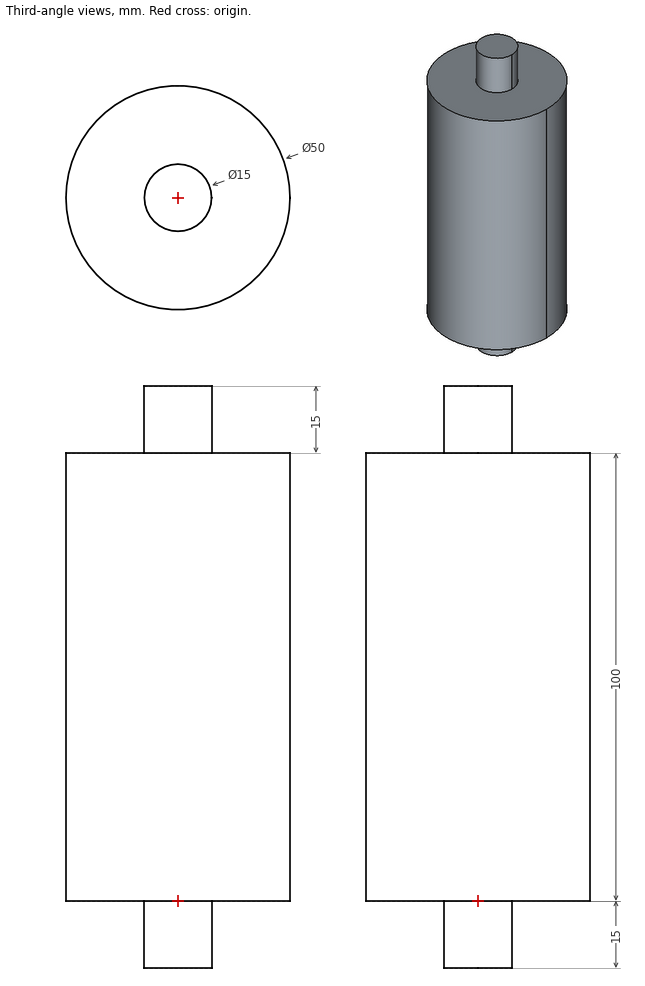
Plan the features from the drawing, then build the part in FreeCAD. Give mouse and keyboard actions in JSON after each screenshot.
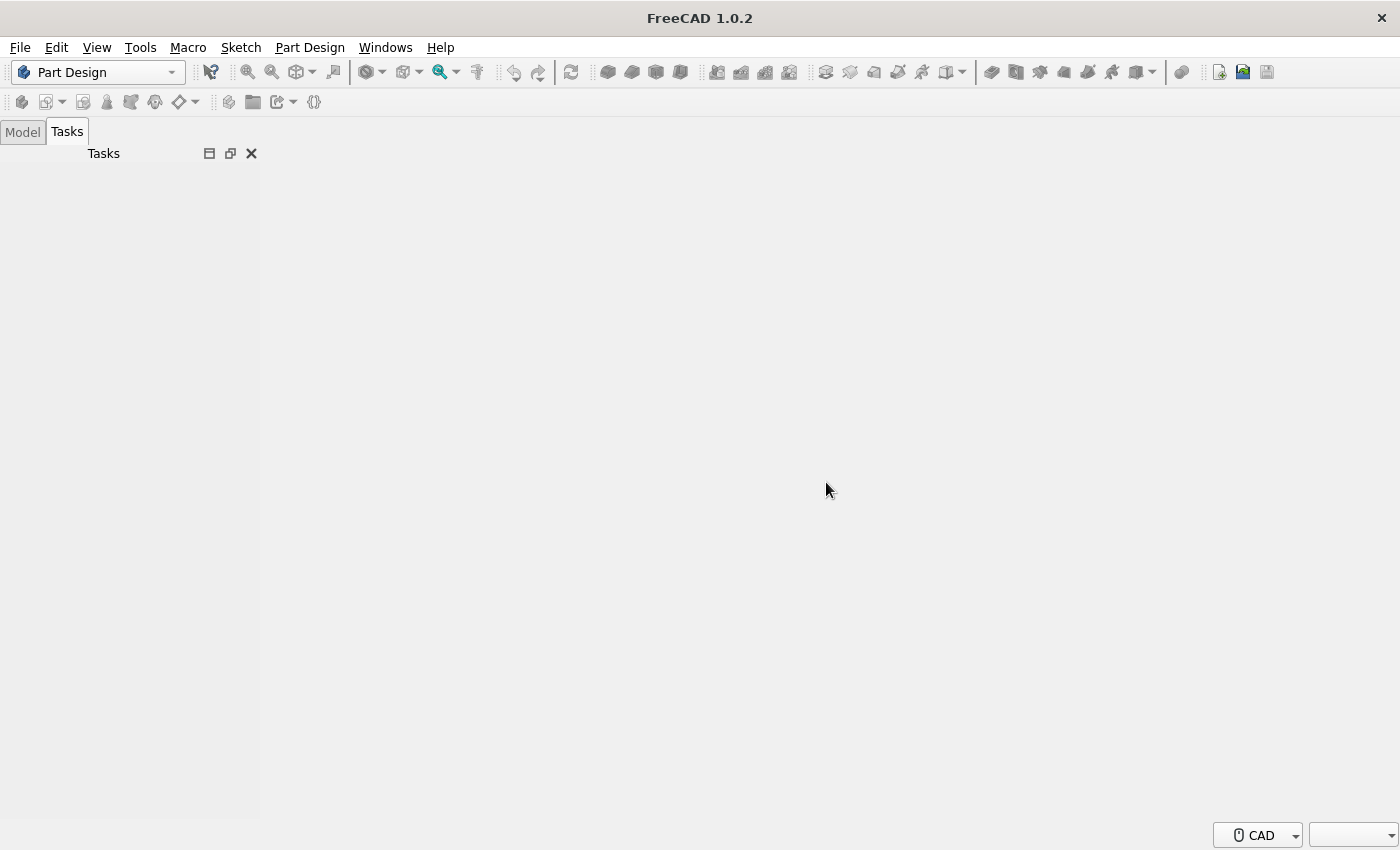
{"action": "left_click", "coordinate": [1220, 72]}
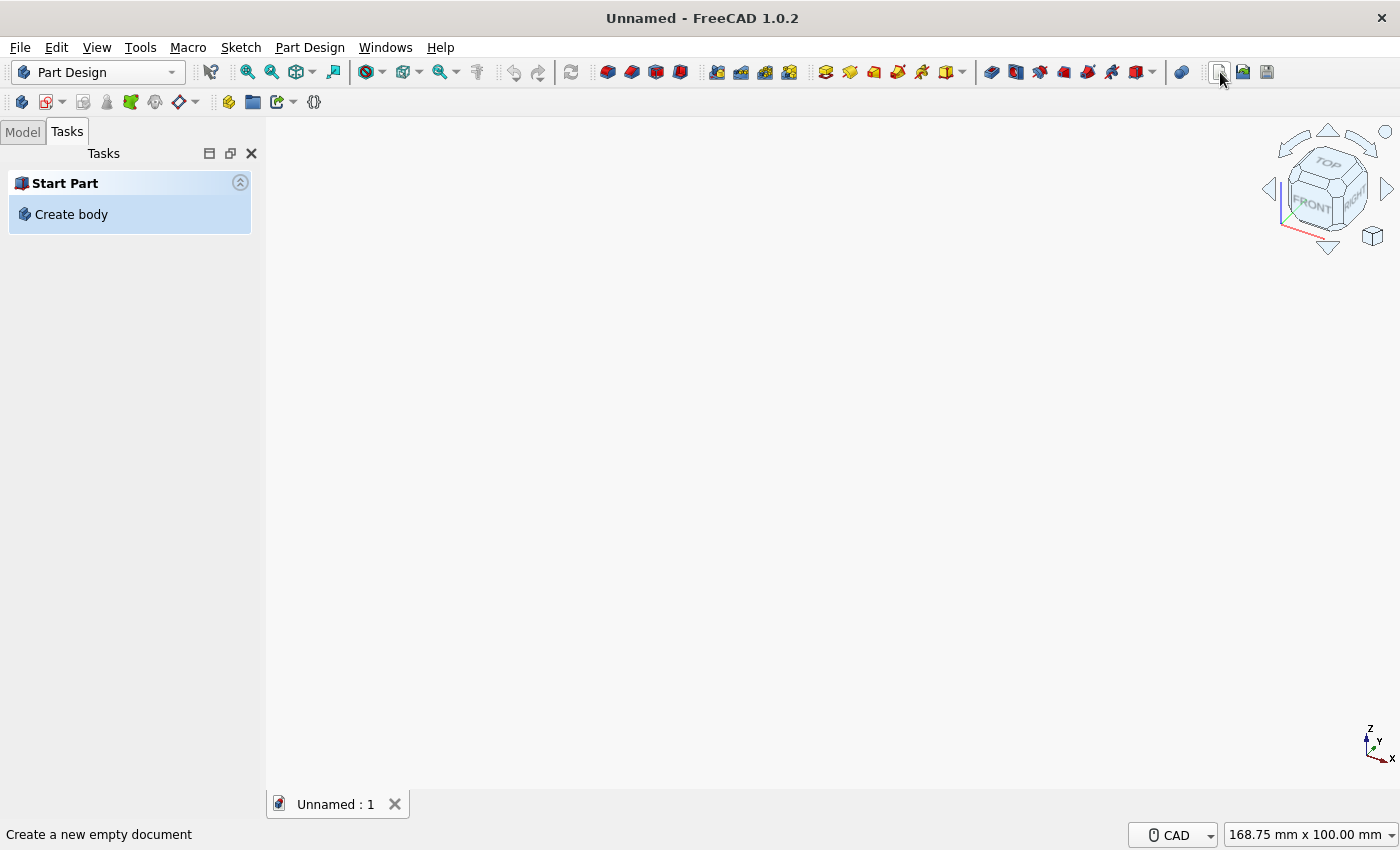
{"action": "left_click", "coordinate": [46, 102]}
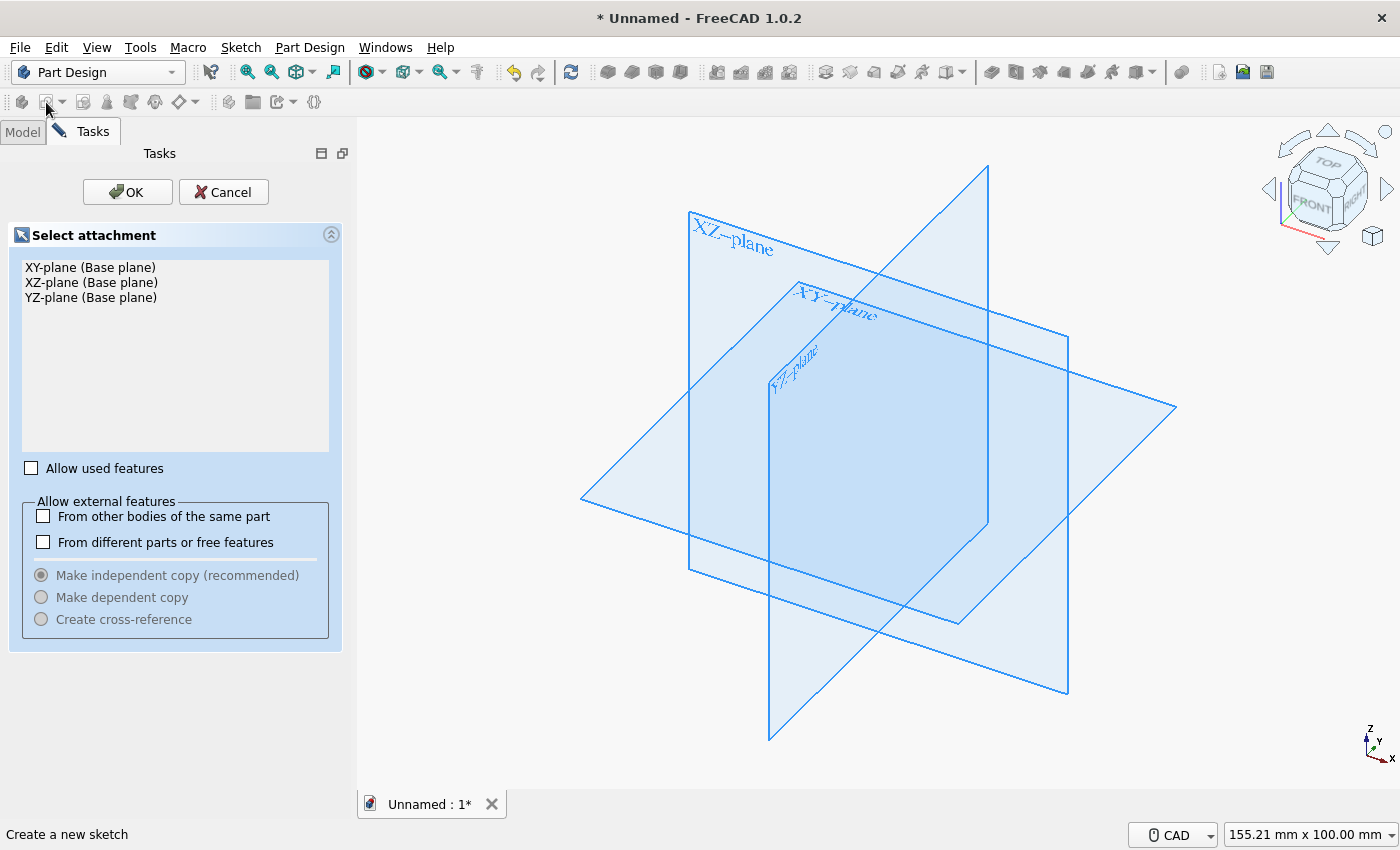
{"action": "left_click", "coordinate": [82, 268]}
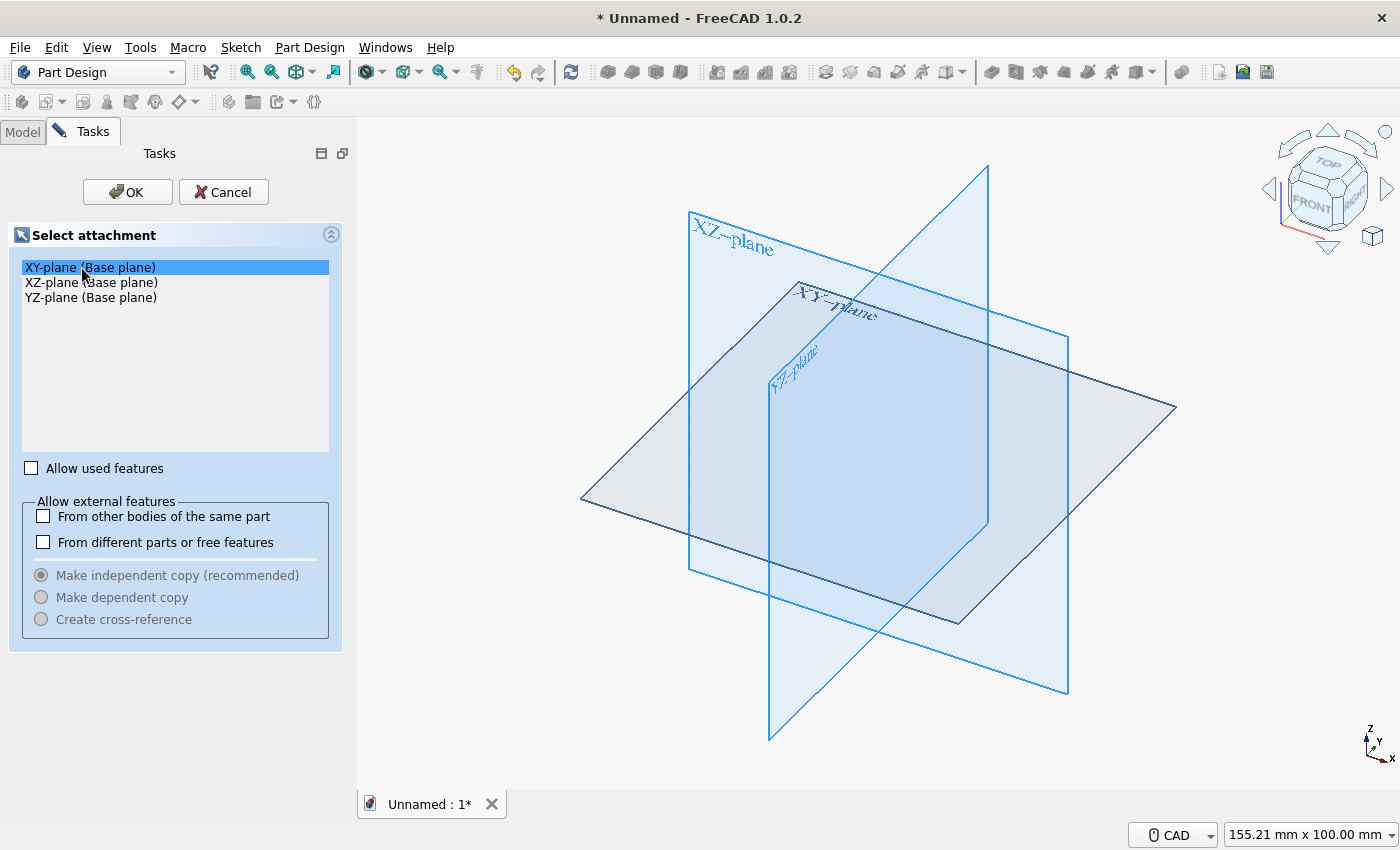
{"action": "left_click", "coordinate": [128, 192]}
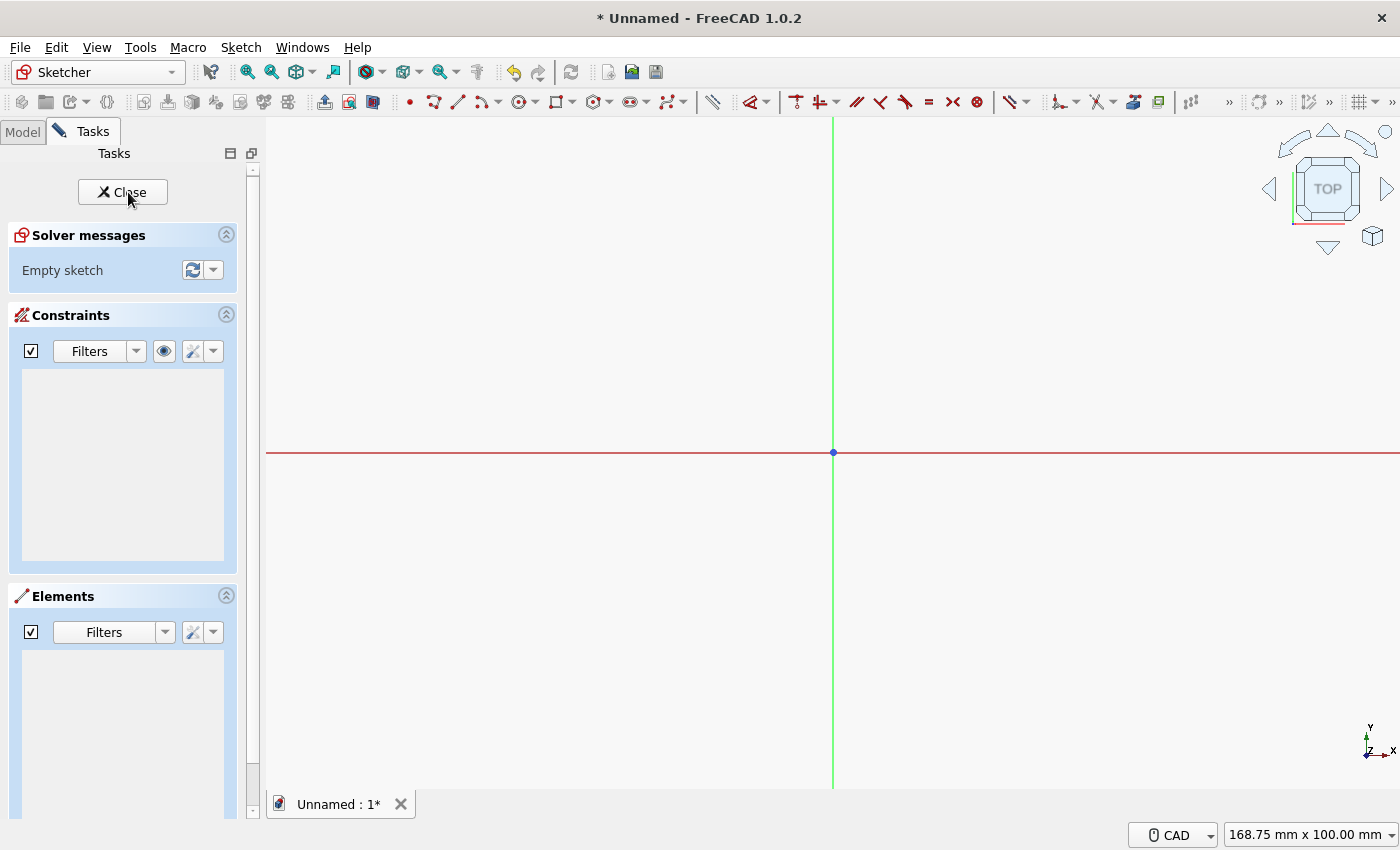
{"action": "left_click", "coordinate": [520, 102]}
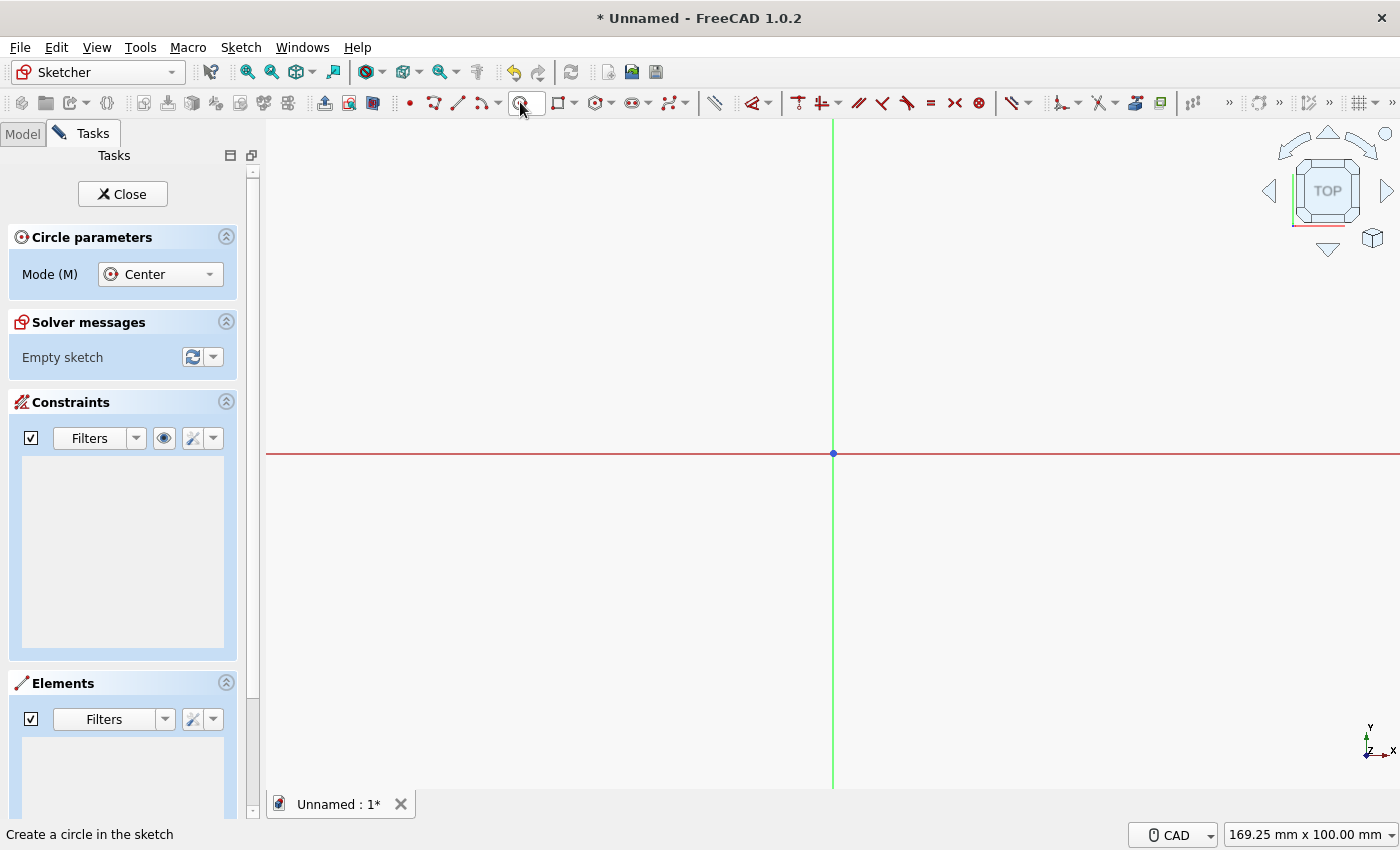
{"action": "left_click", "coordinate": [833, 454]}
{"action": "left_click", "coordinate": [951, 336]}
{"action": "key", "text": "Escape"}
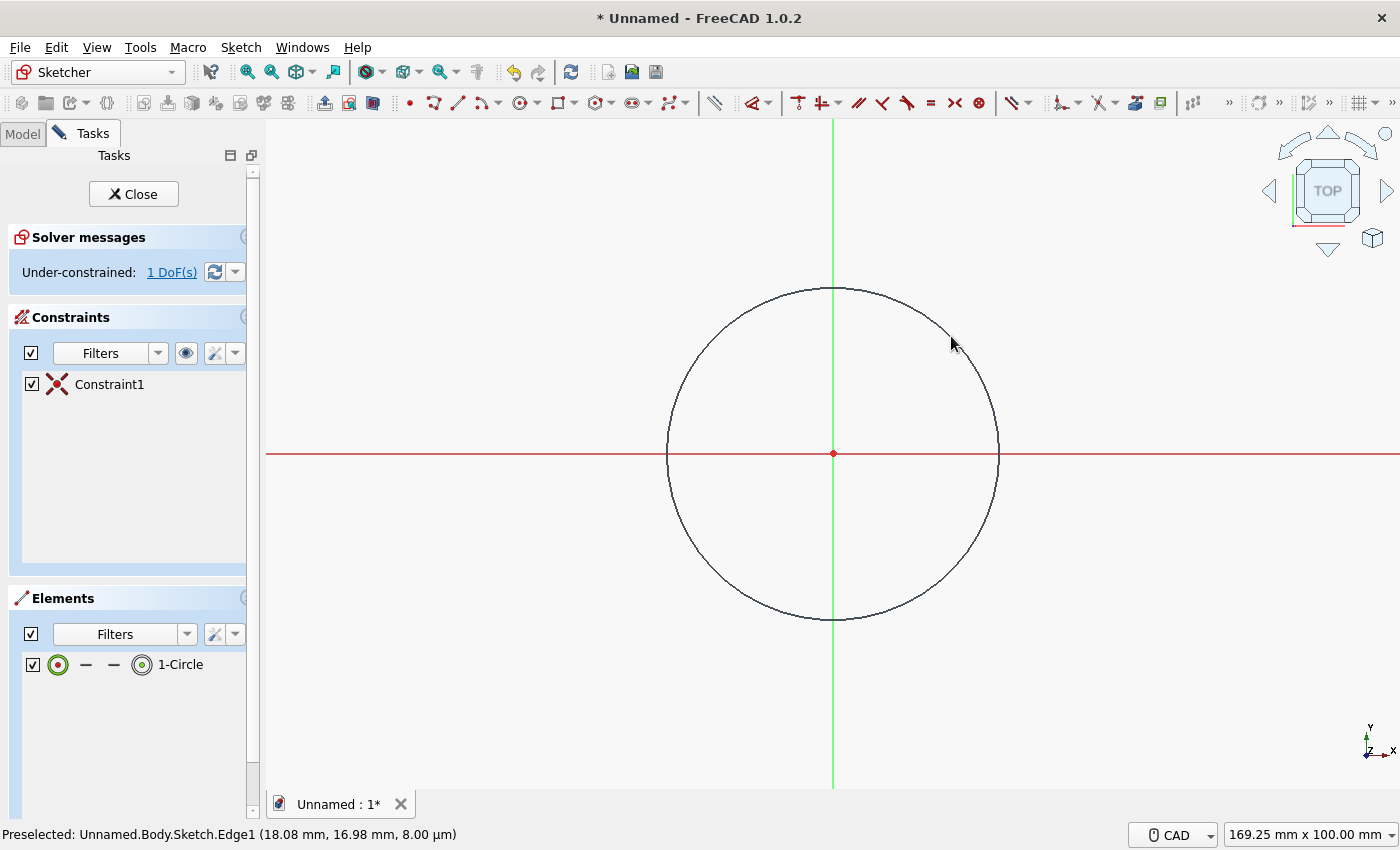
{"action": "left_click", "coordinate": [752, 104]}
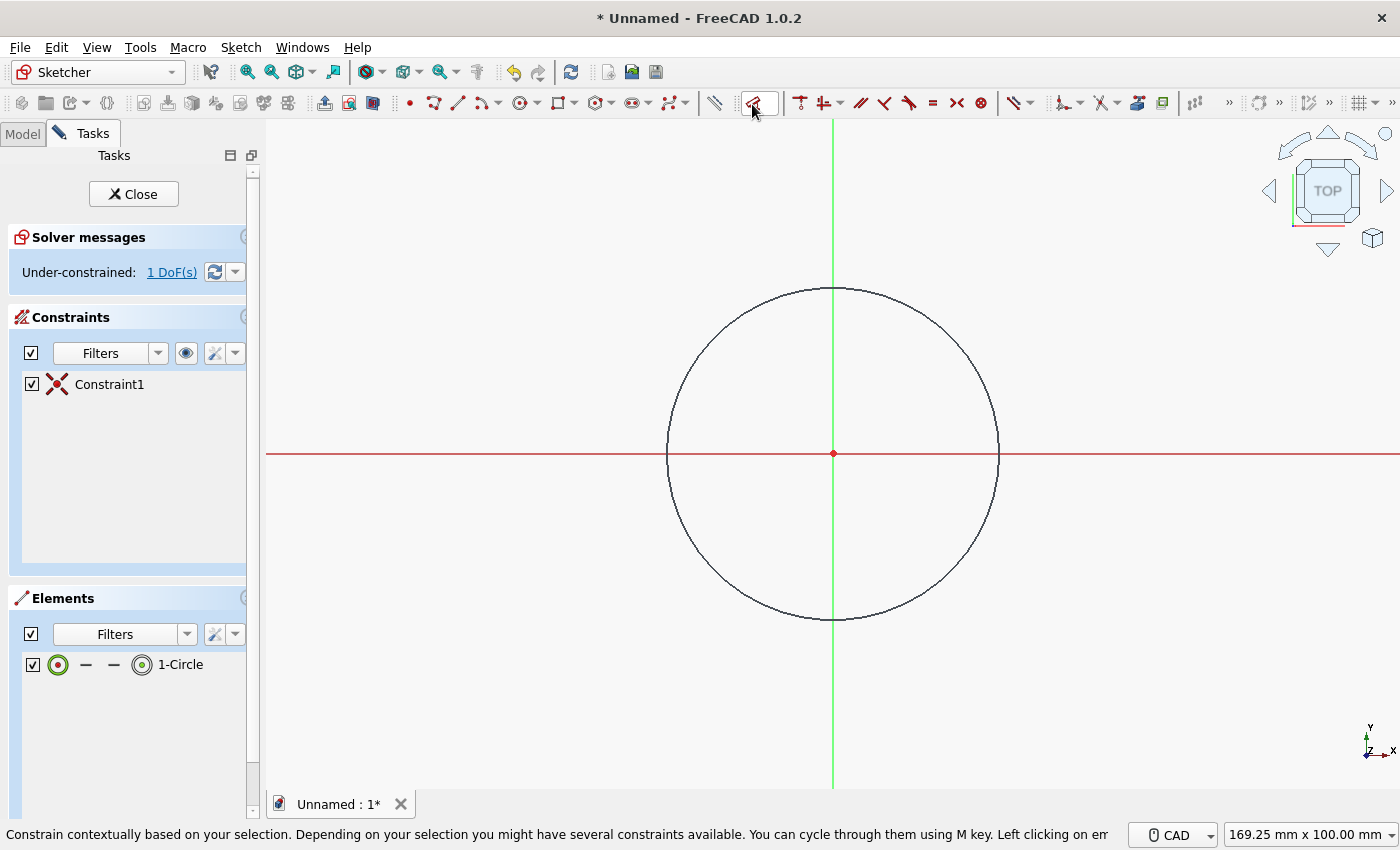
{"action": "left_click", "coordinate": [950, 336]}
{"action": "left_click", "coordinate": [973, 313]}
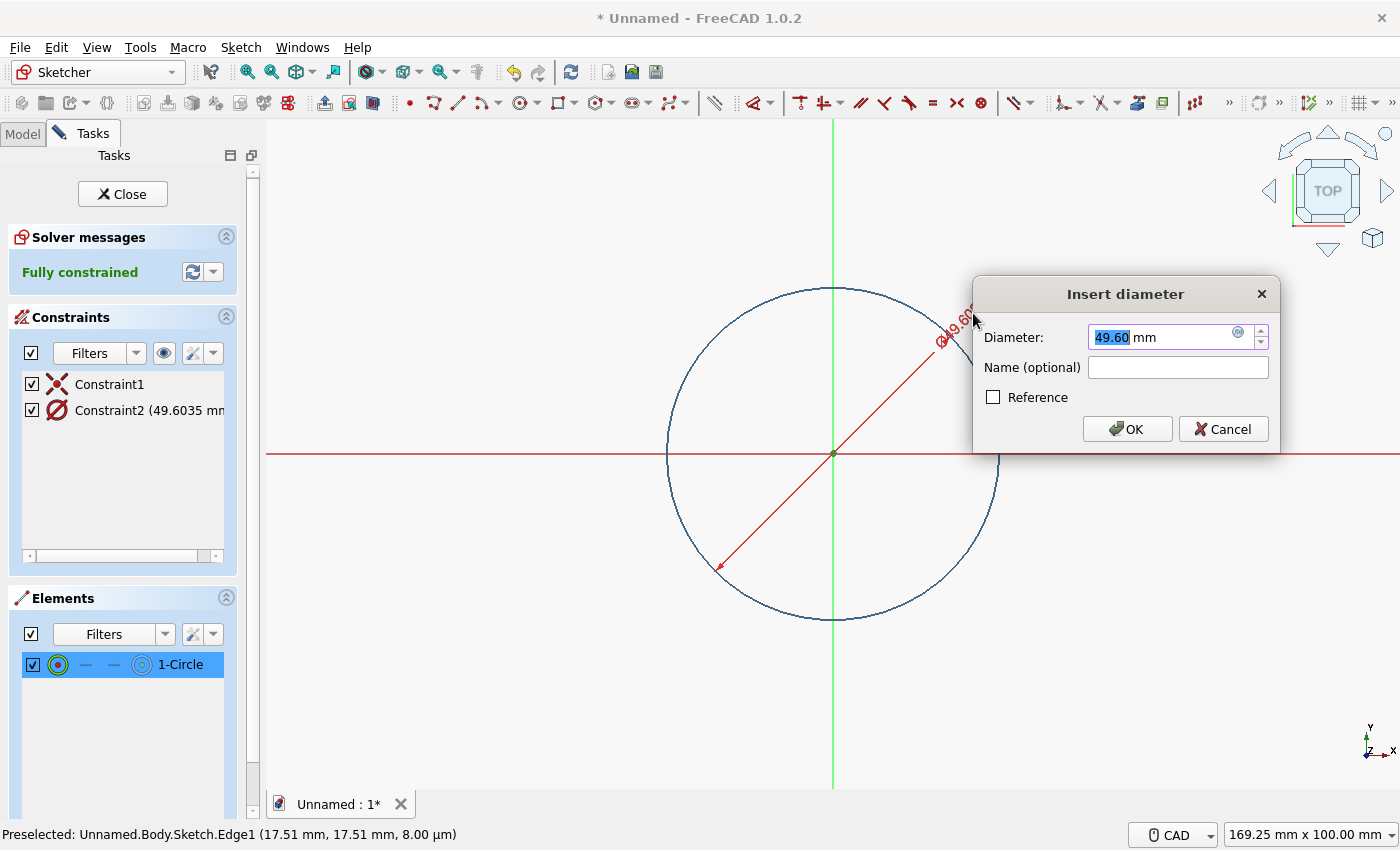
{"action": "type", "text": "50"}
{"action": "key", "text": "Return"}
{"action": "key", "text": "Escape"}